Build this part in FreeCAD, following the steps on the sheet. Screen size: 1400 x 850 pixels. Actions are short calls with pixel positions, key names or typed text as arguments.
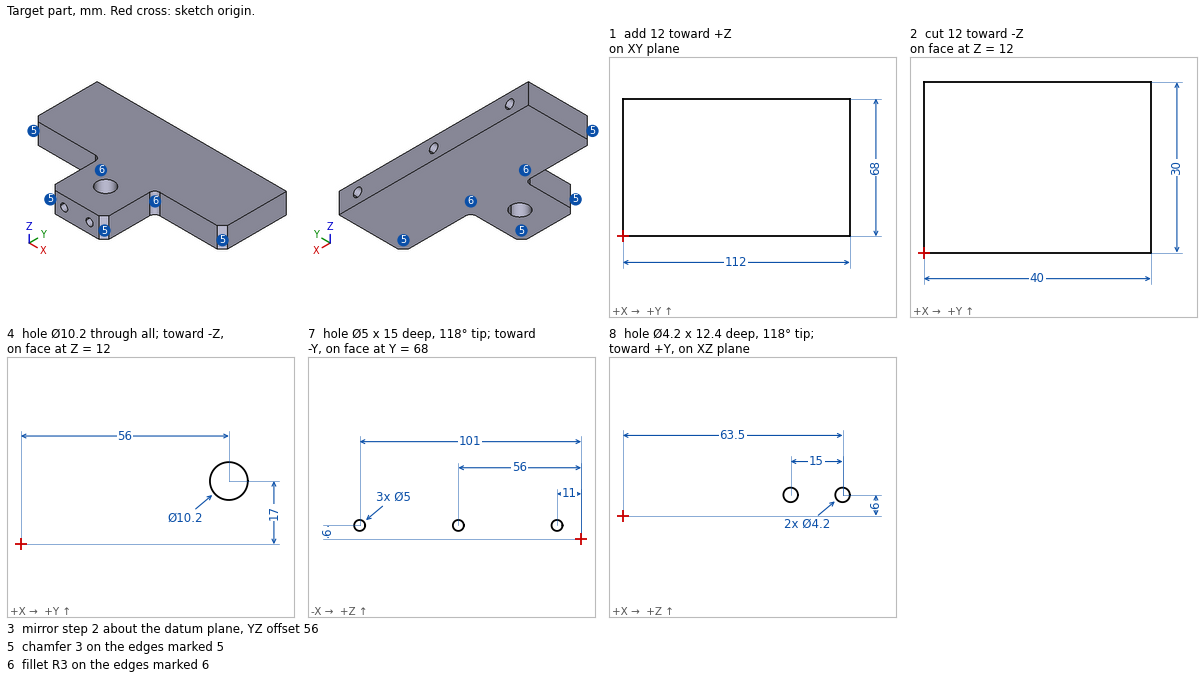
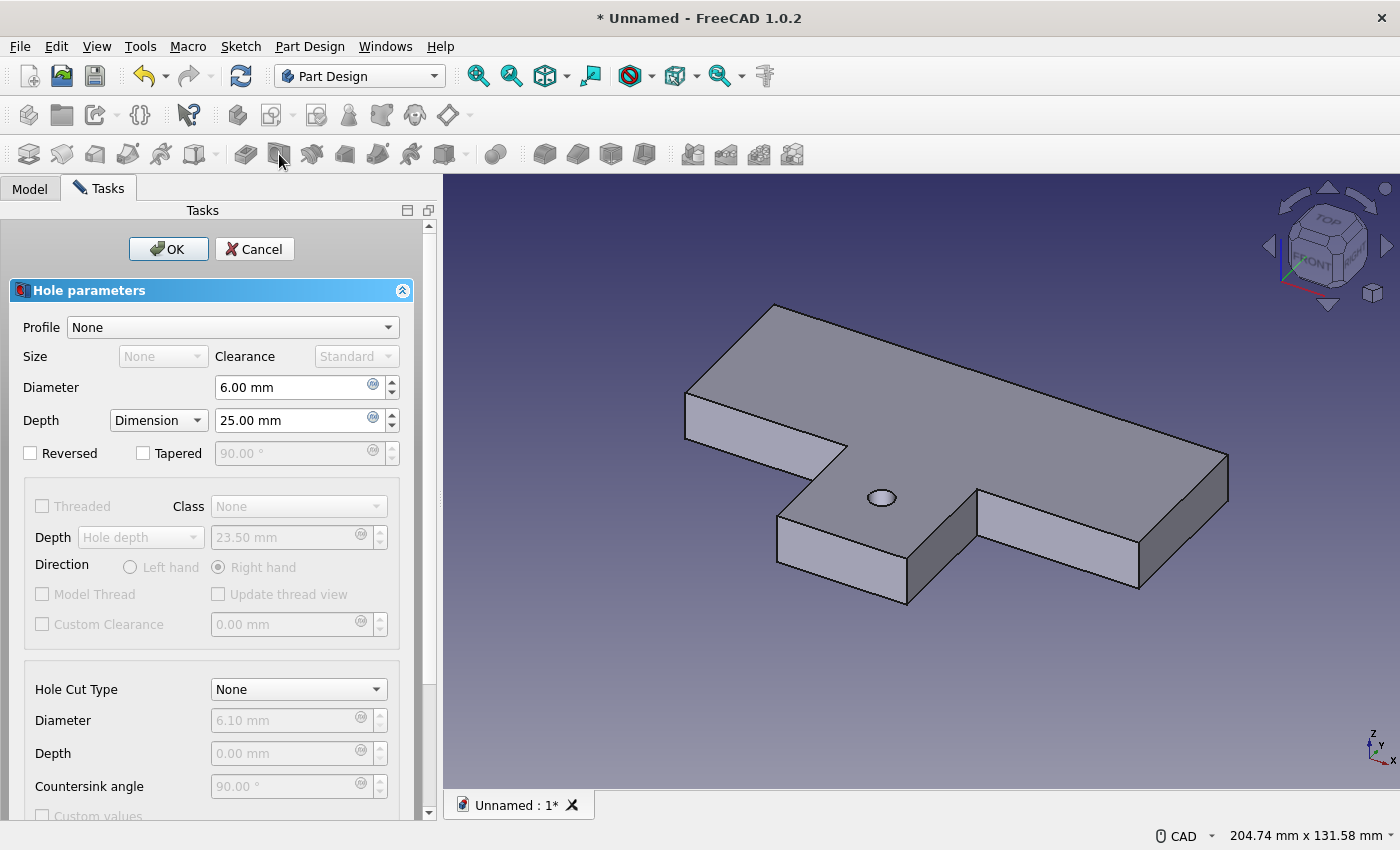
triple_click(300, 388)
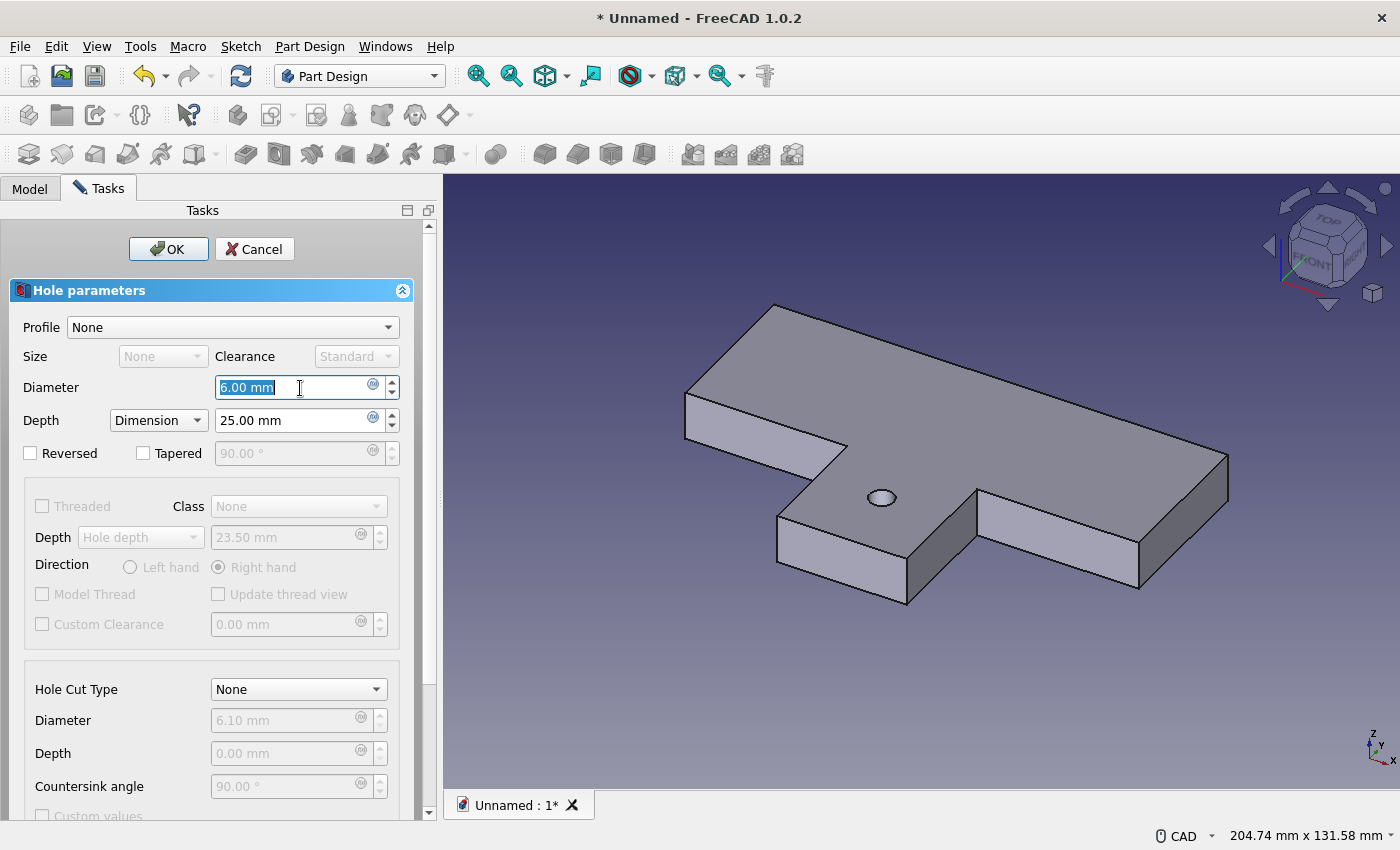
text(10.2)
key(Tab)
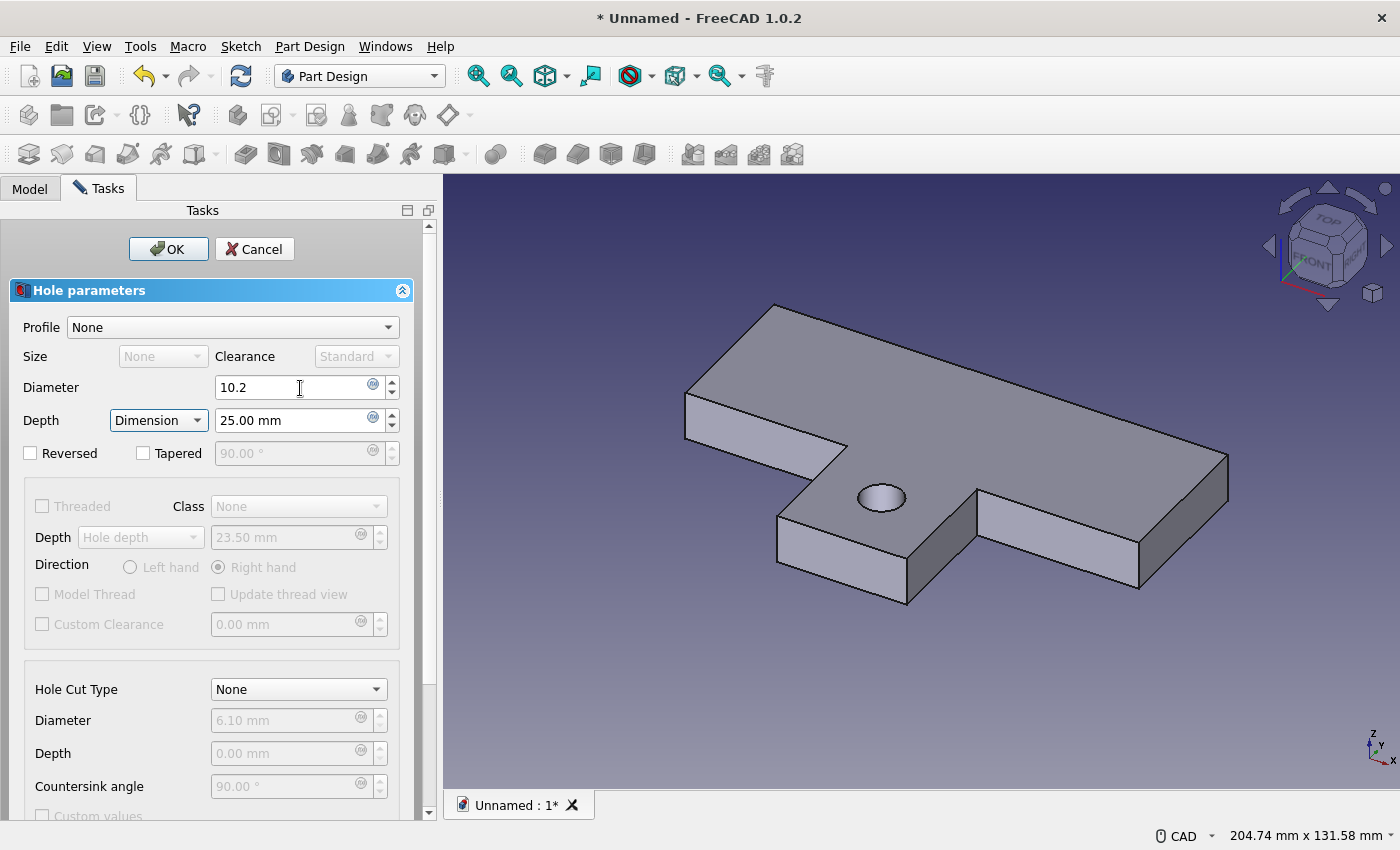
click(160, 420)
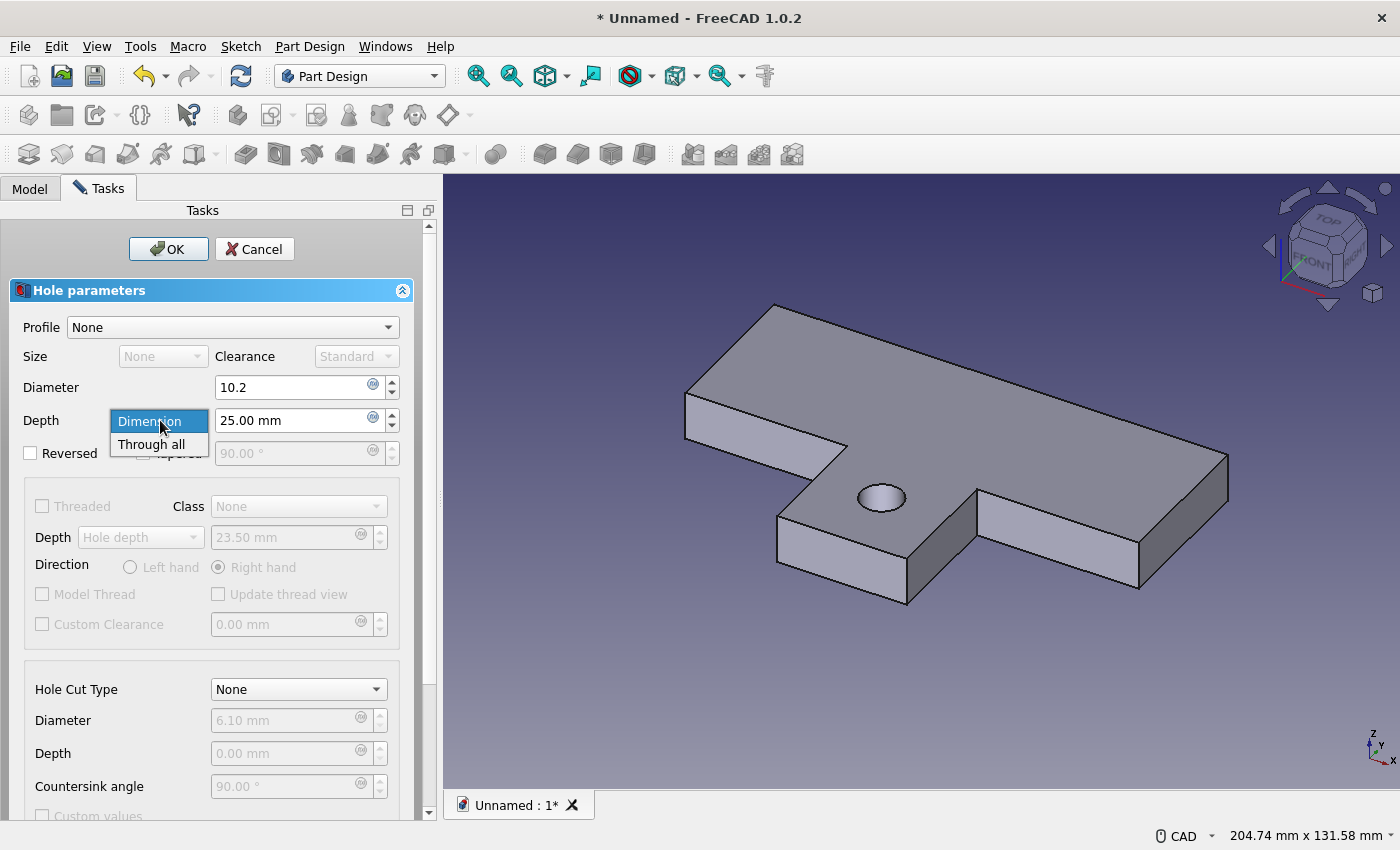
click(158, 444)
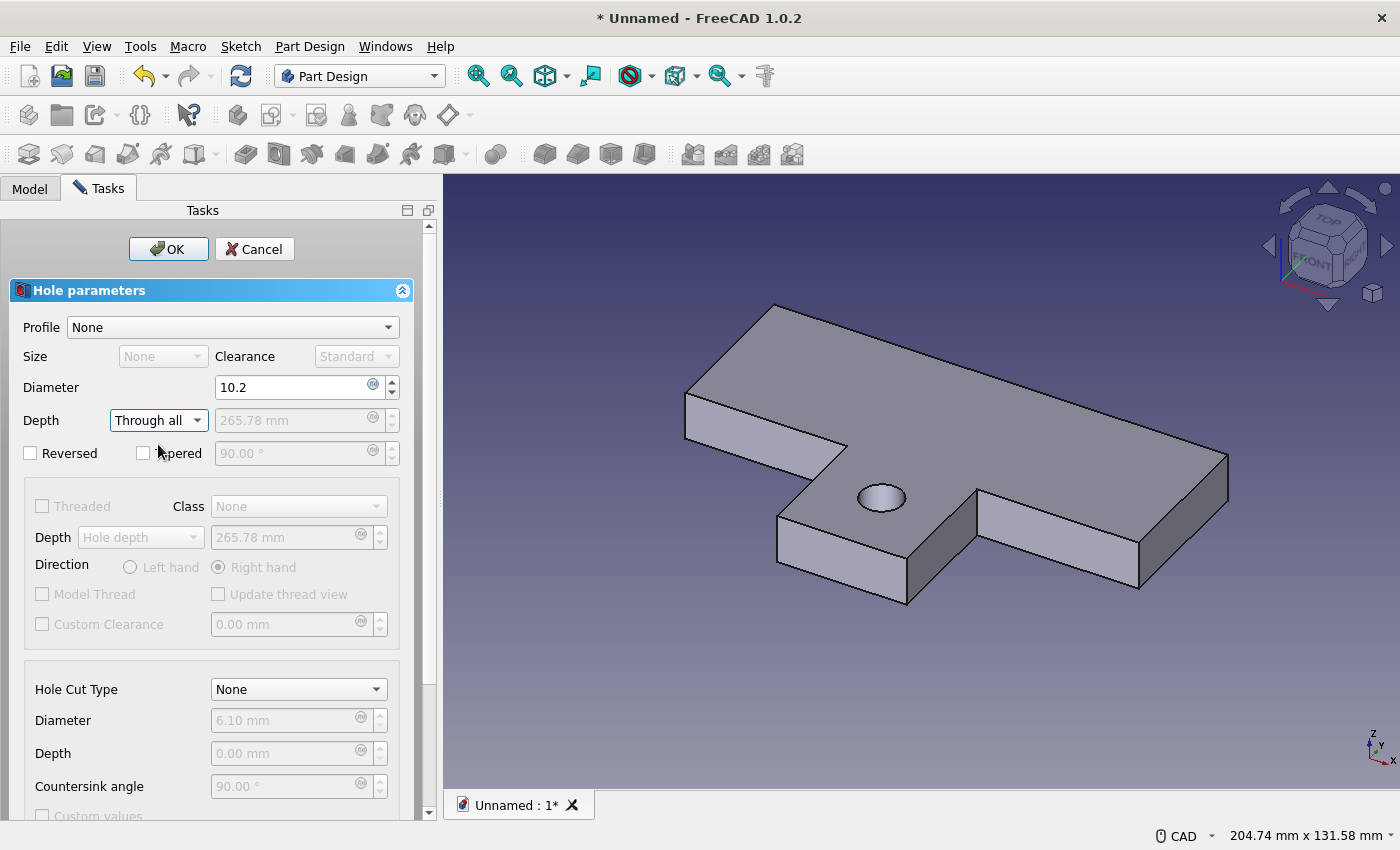
click(169, 249)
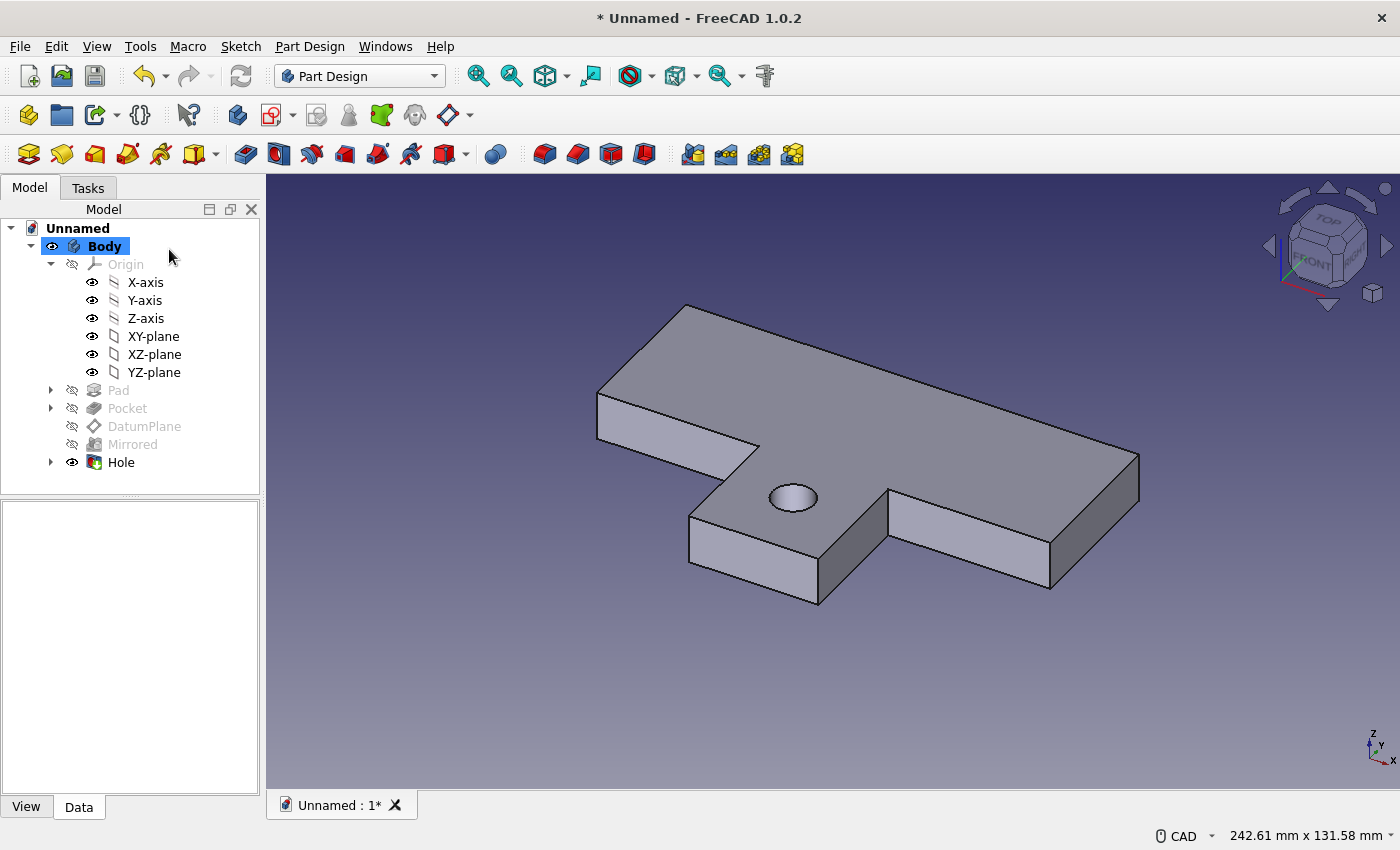
click(1050, 565)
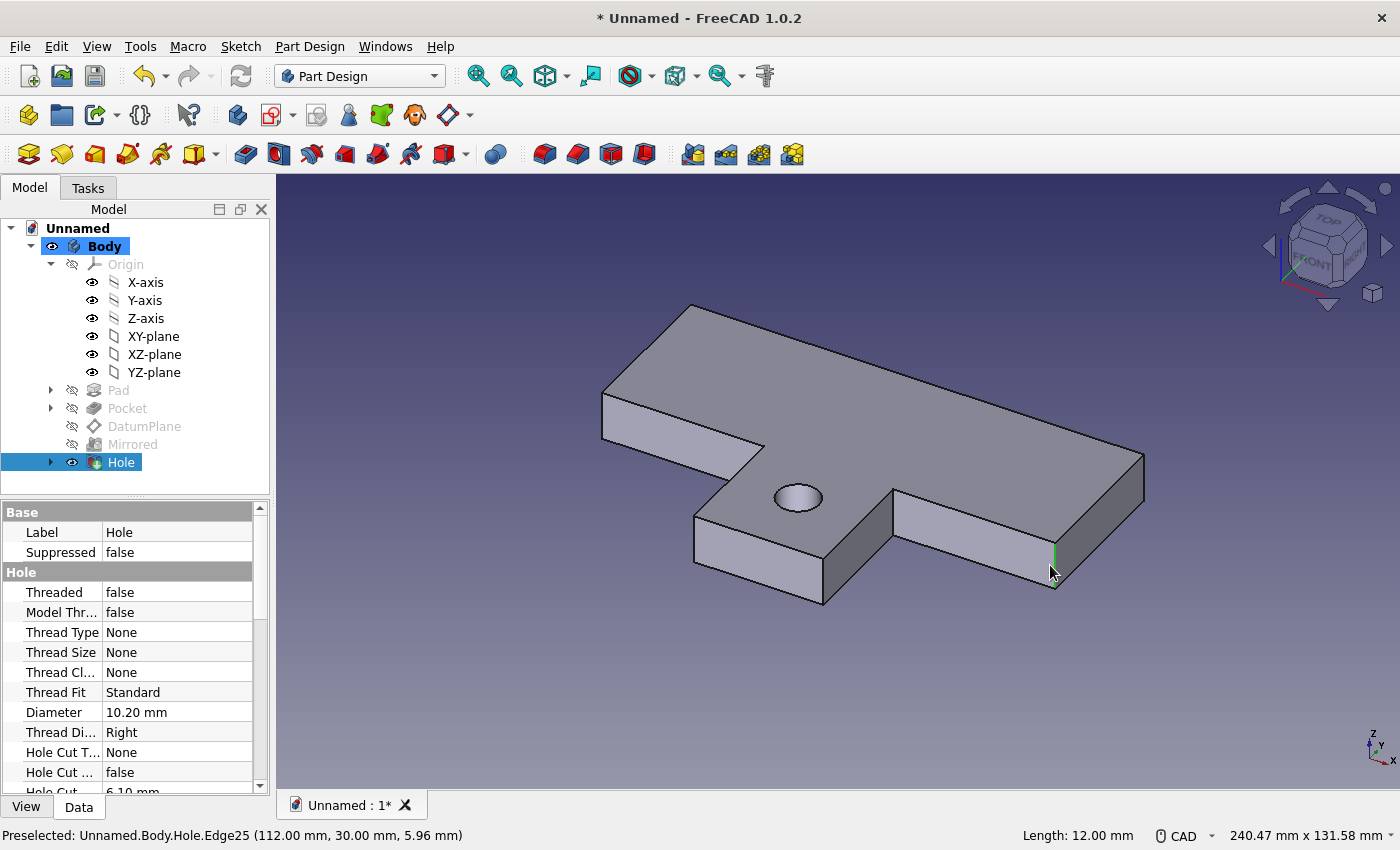
click(823, 581, ctrl)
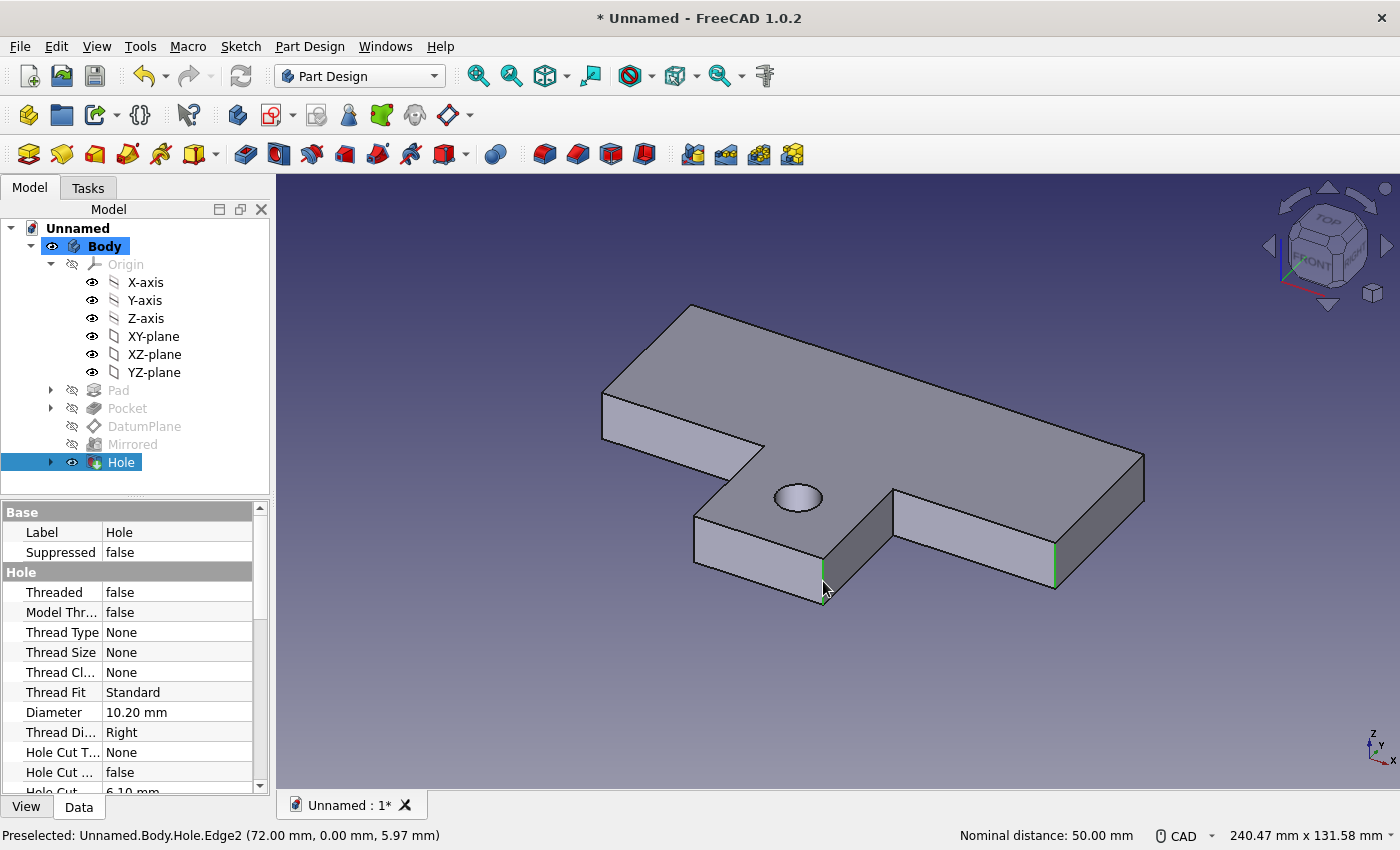
key(0)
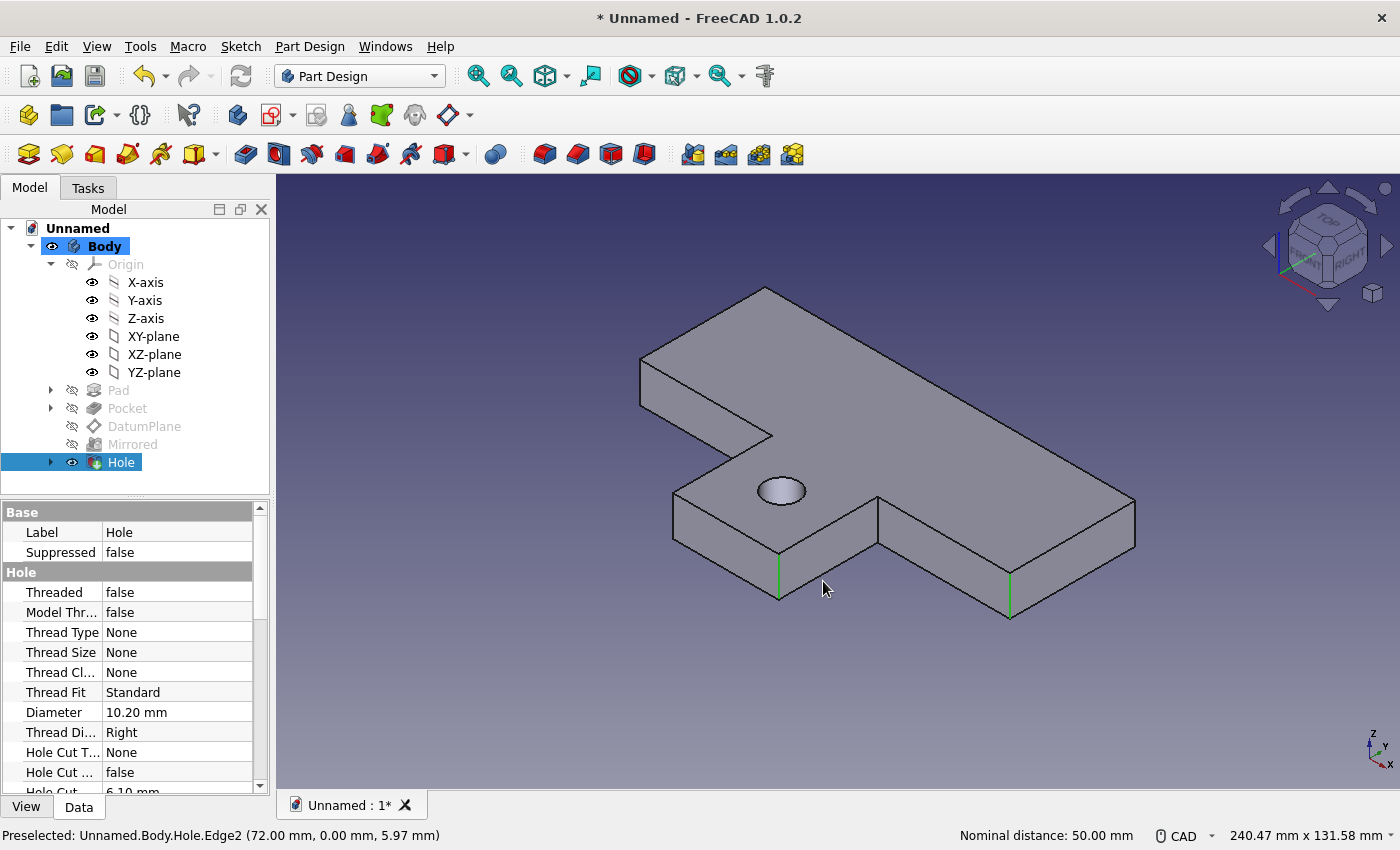
key(2)